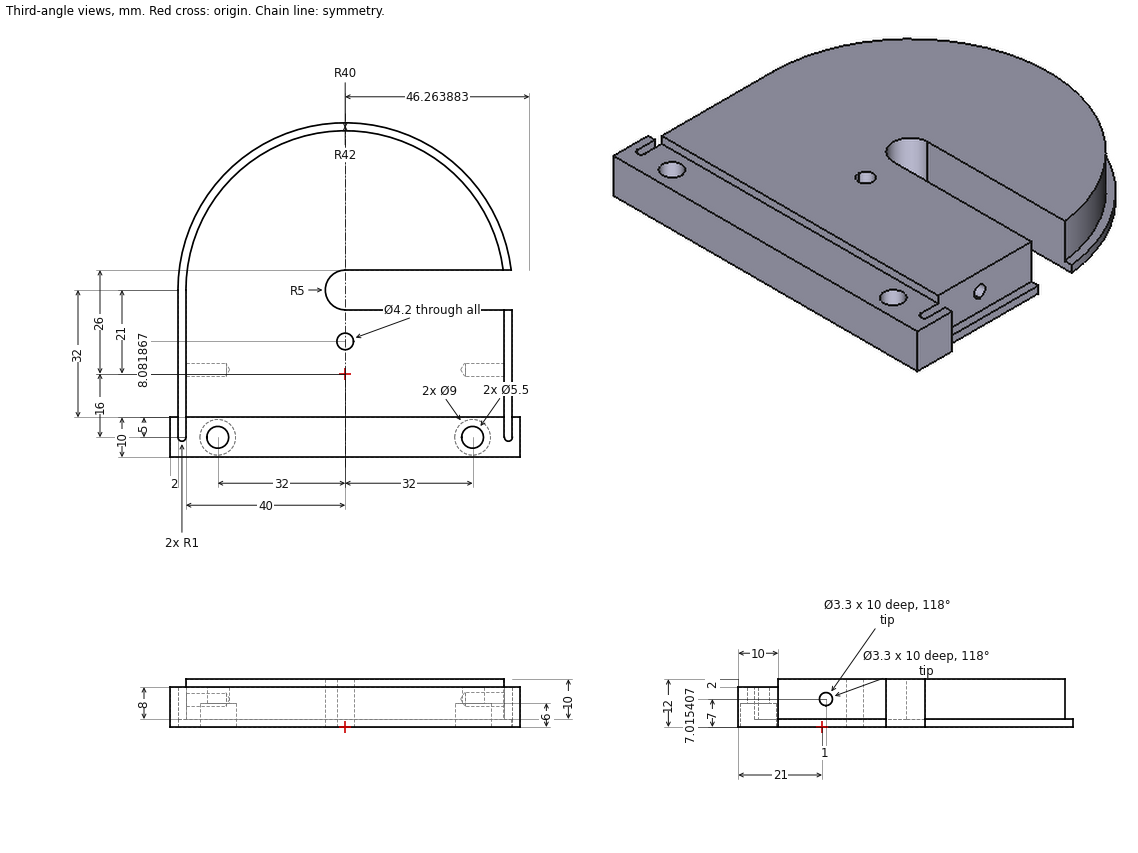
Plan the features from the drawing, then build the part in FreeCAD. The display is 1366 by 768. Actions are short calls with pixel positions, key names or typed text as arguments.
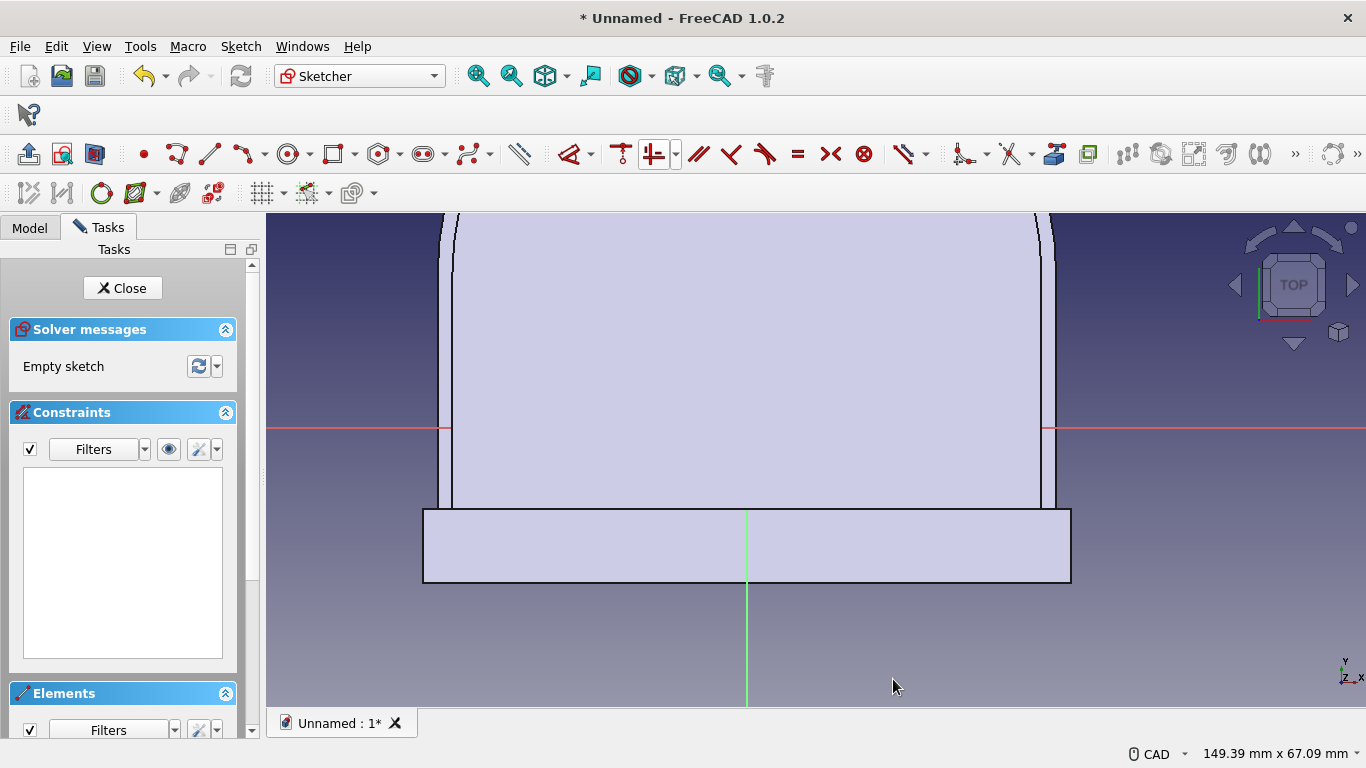
click(177, 154)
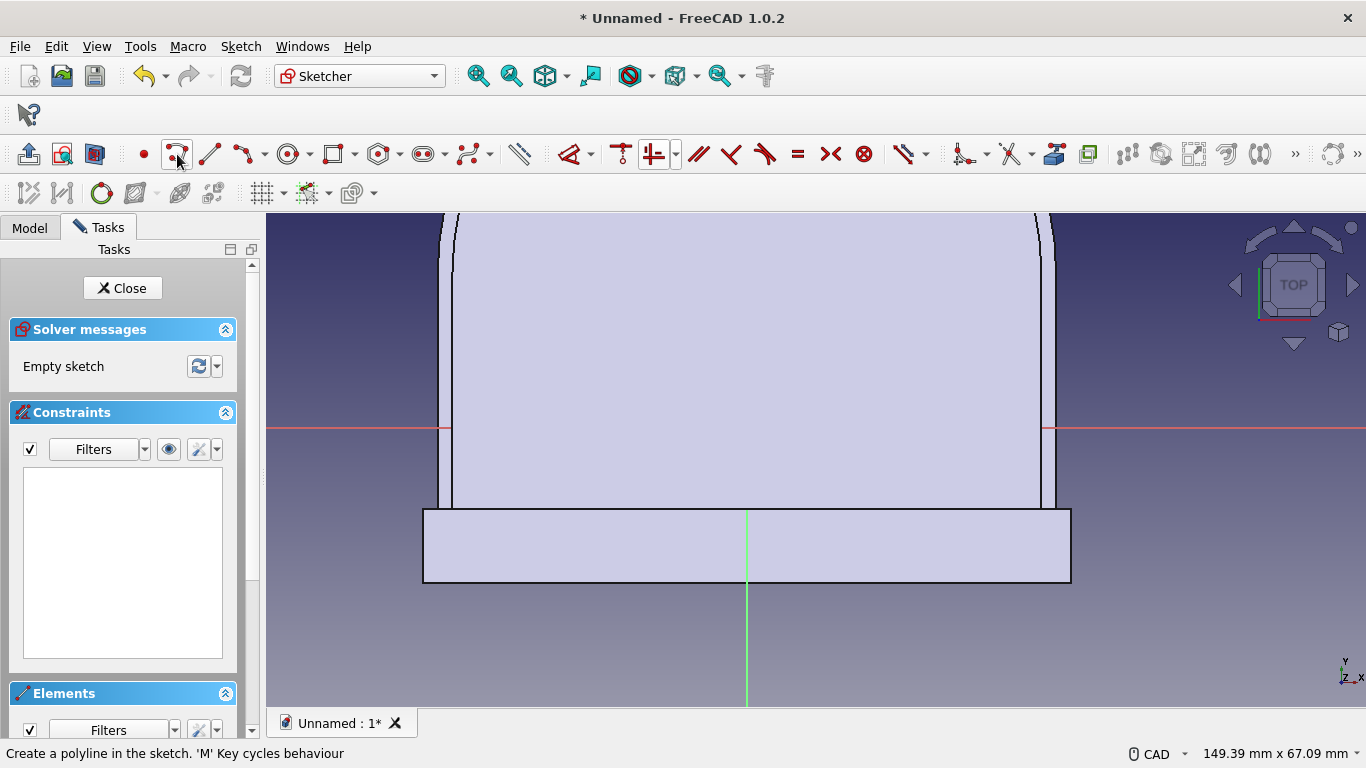
click(452, 546)
click(452, 509)
click(438, 509)
click(438, 546)
right_click(438, 546)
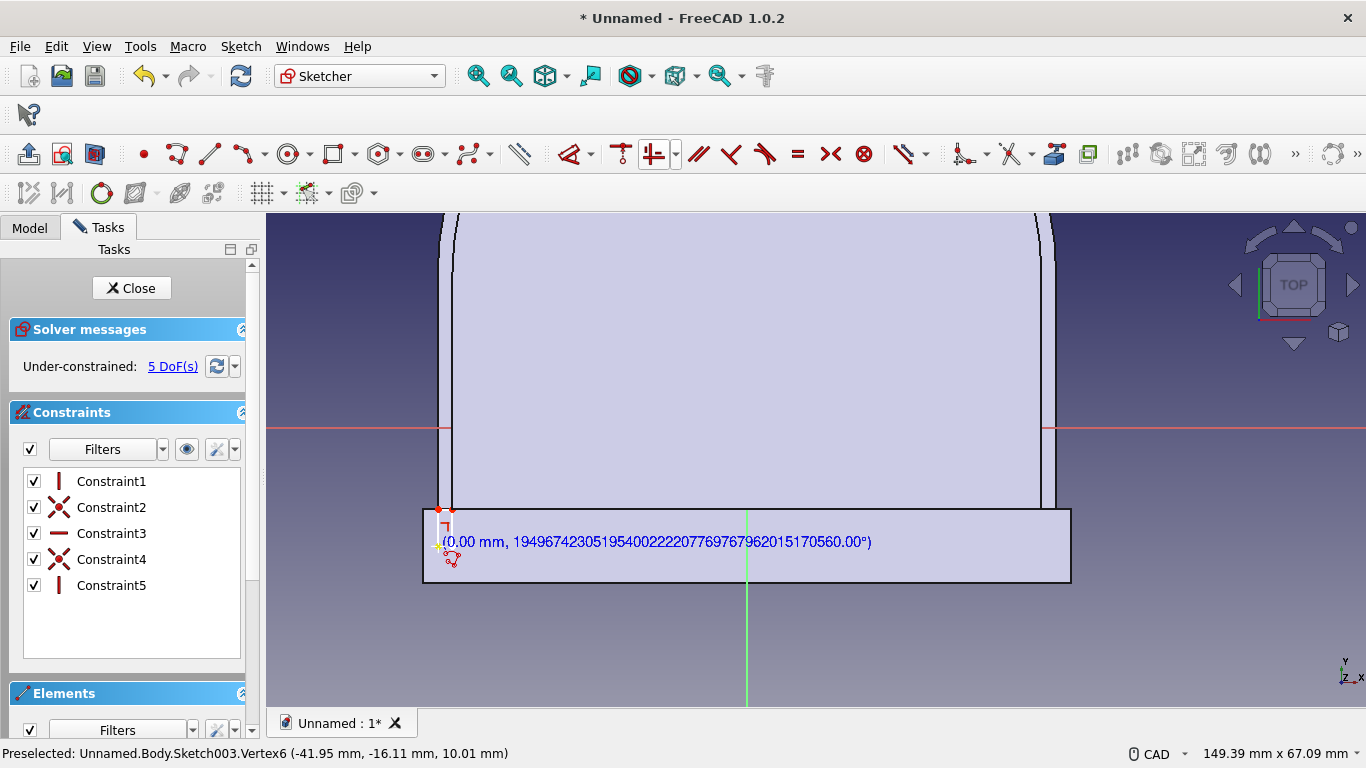
click(242, 154)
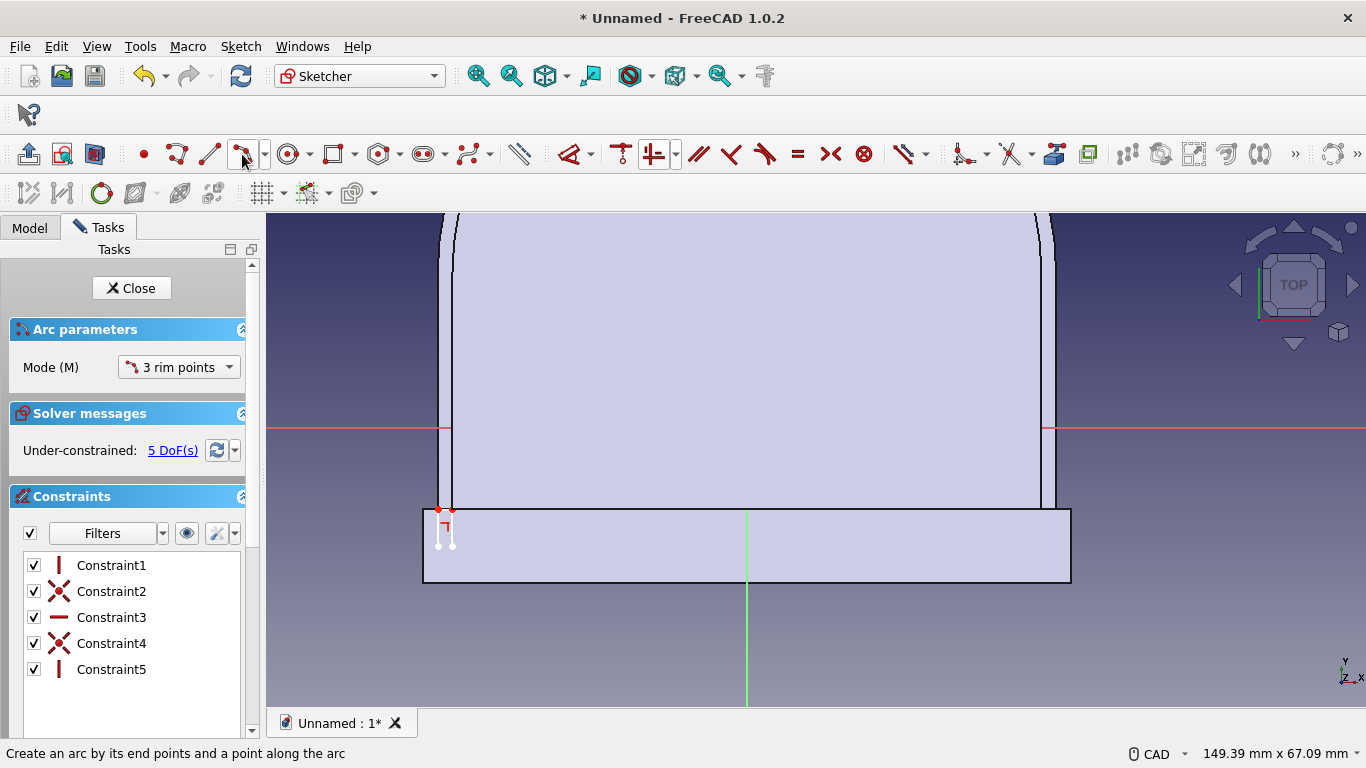
click(438, 547)
click(452, 547)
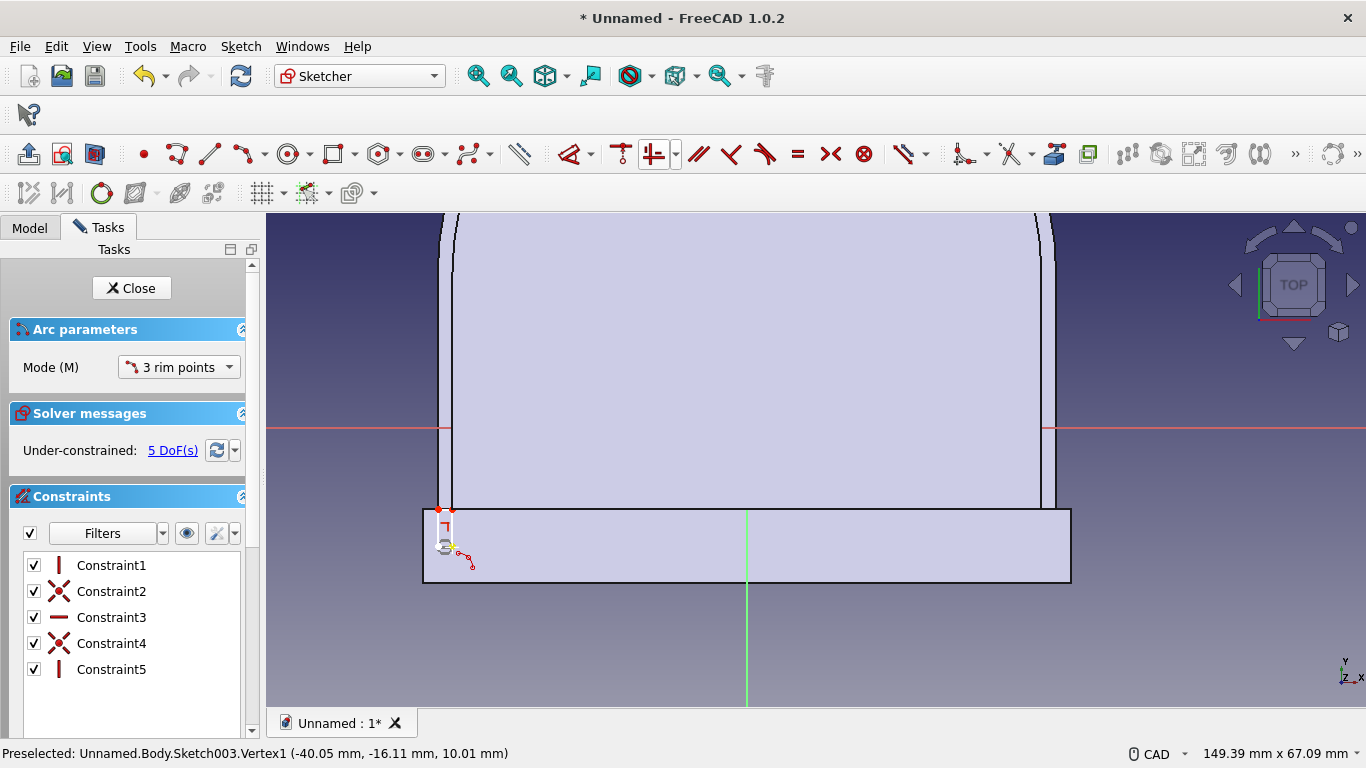
scroll(445, 554, up, 4)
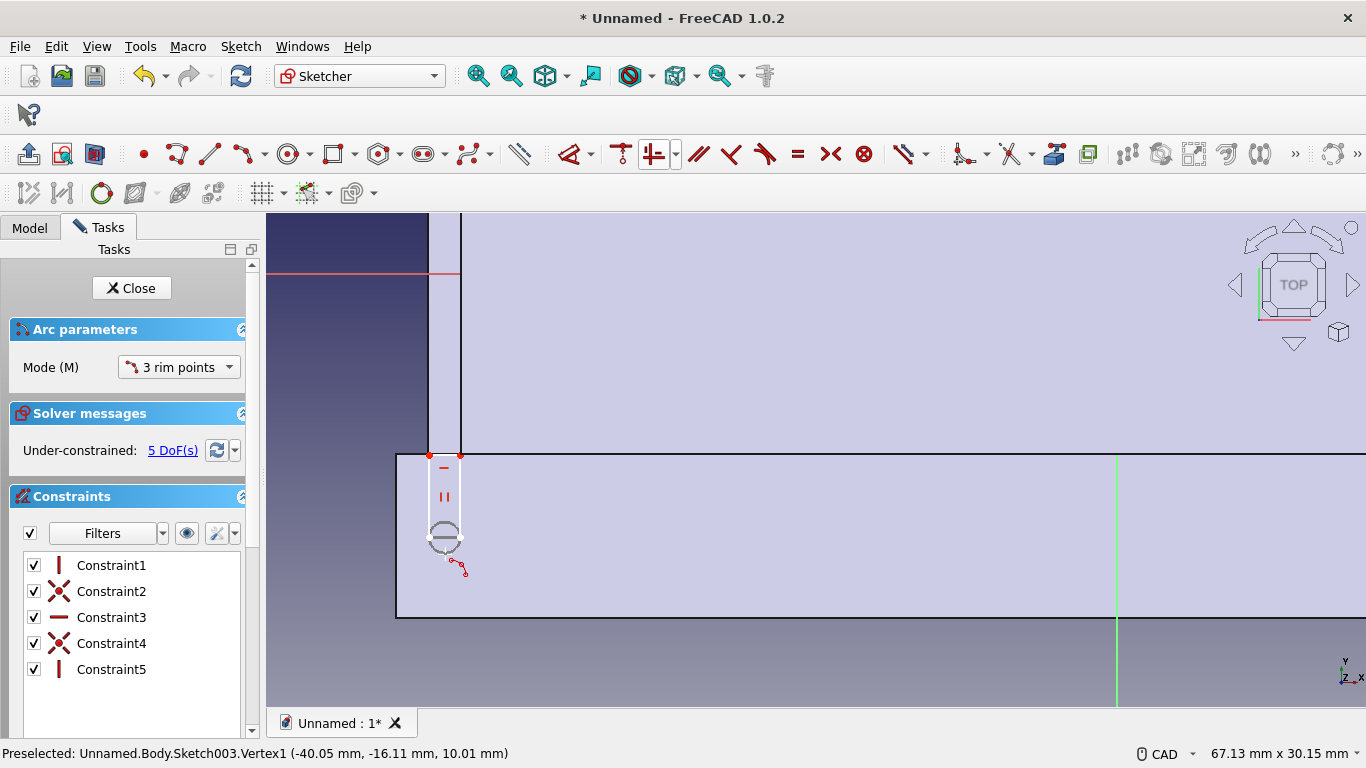
click(445, 552)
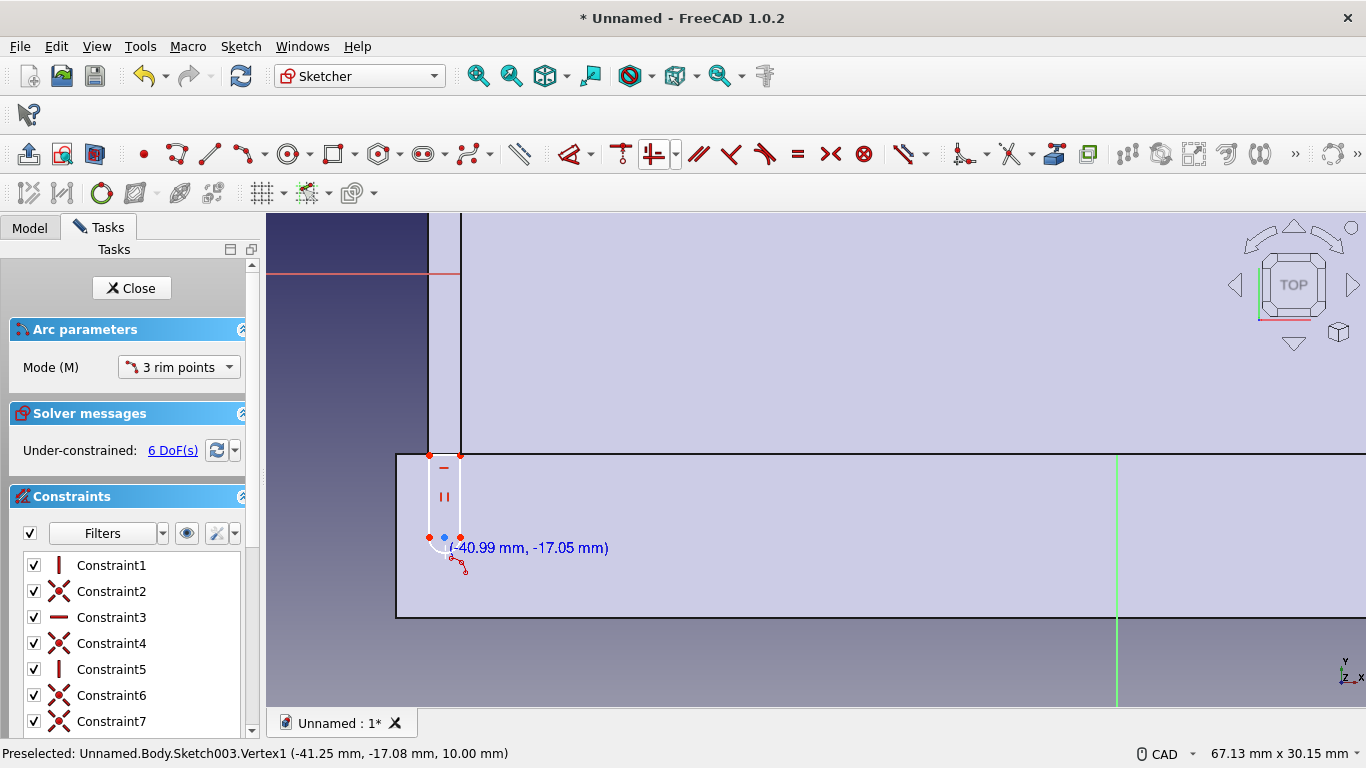
click(177, 154)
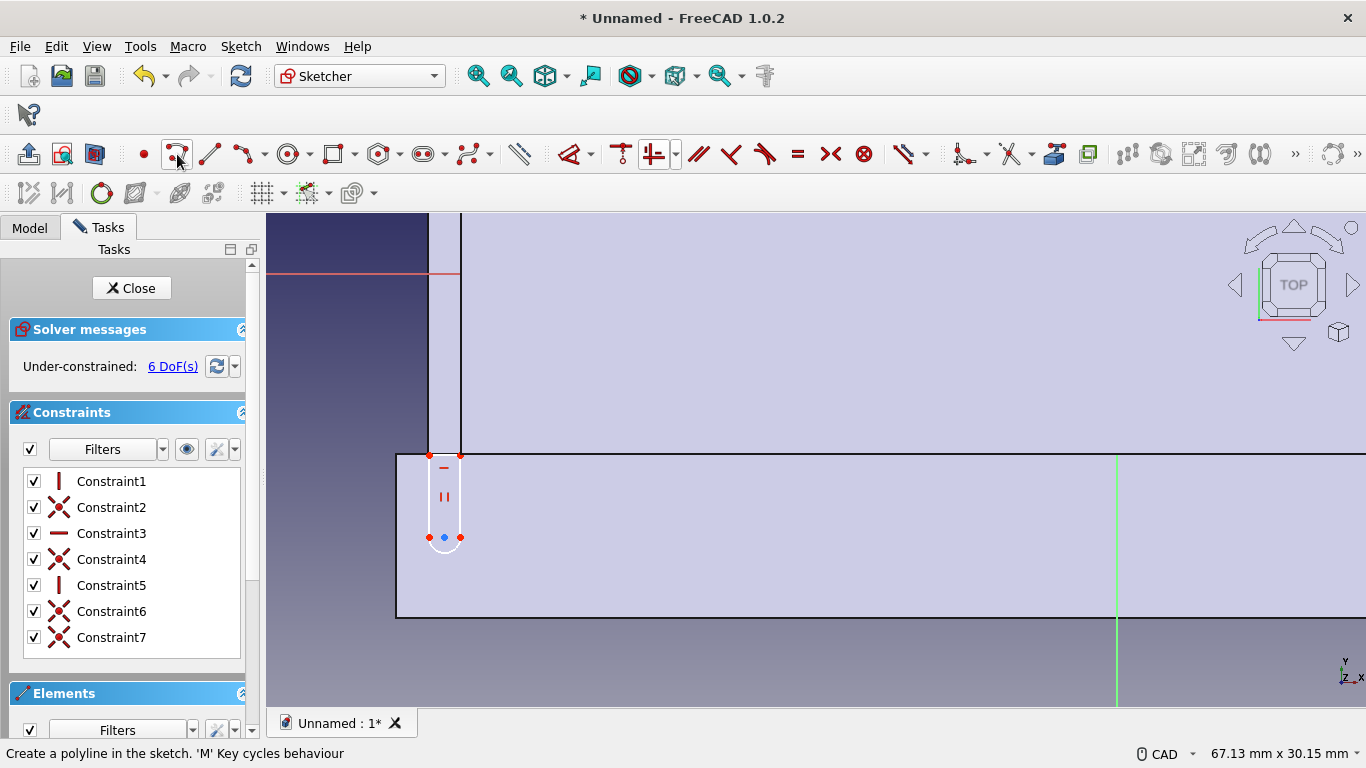
scroll(446, 498, down, 4)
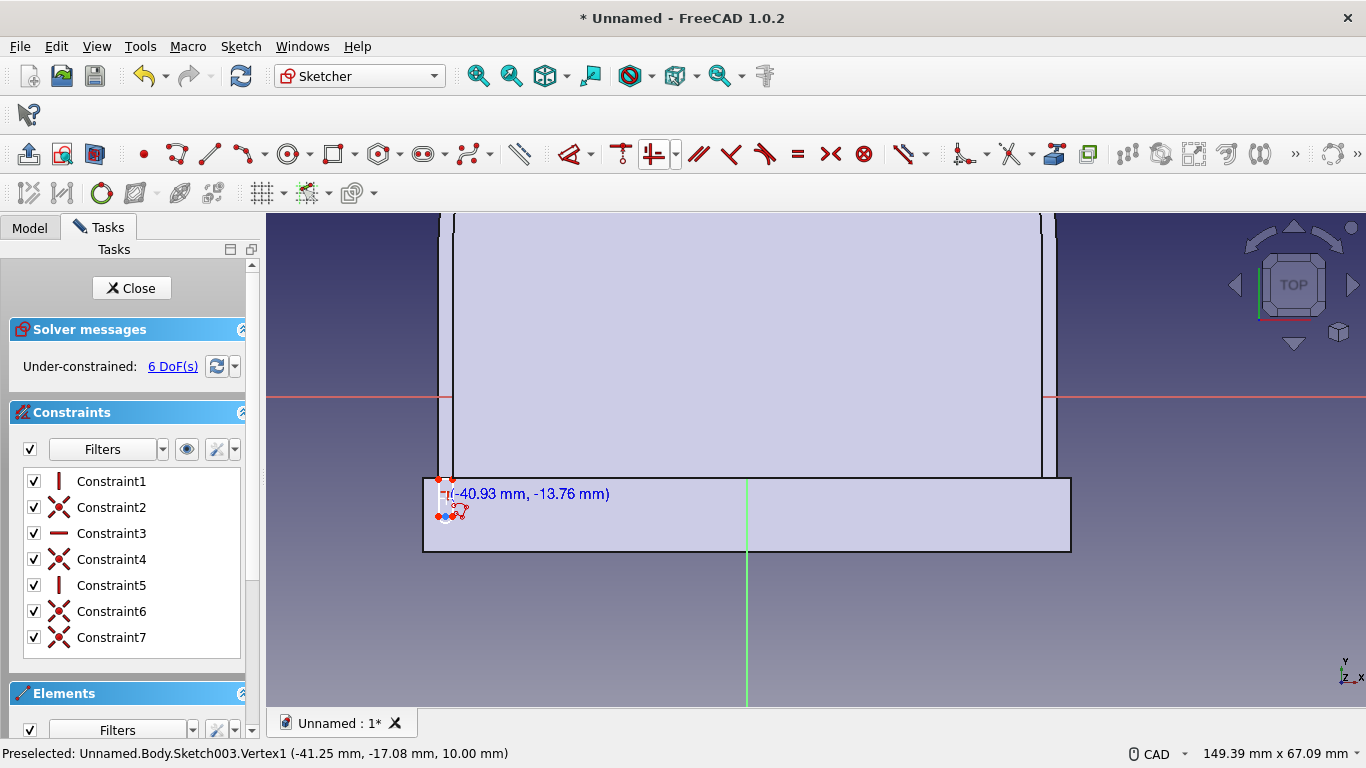
click(1057, 515)
click(1057, 478)
click(1042, 478)
click(1042, 515)
right_click(1042, 515)